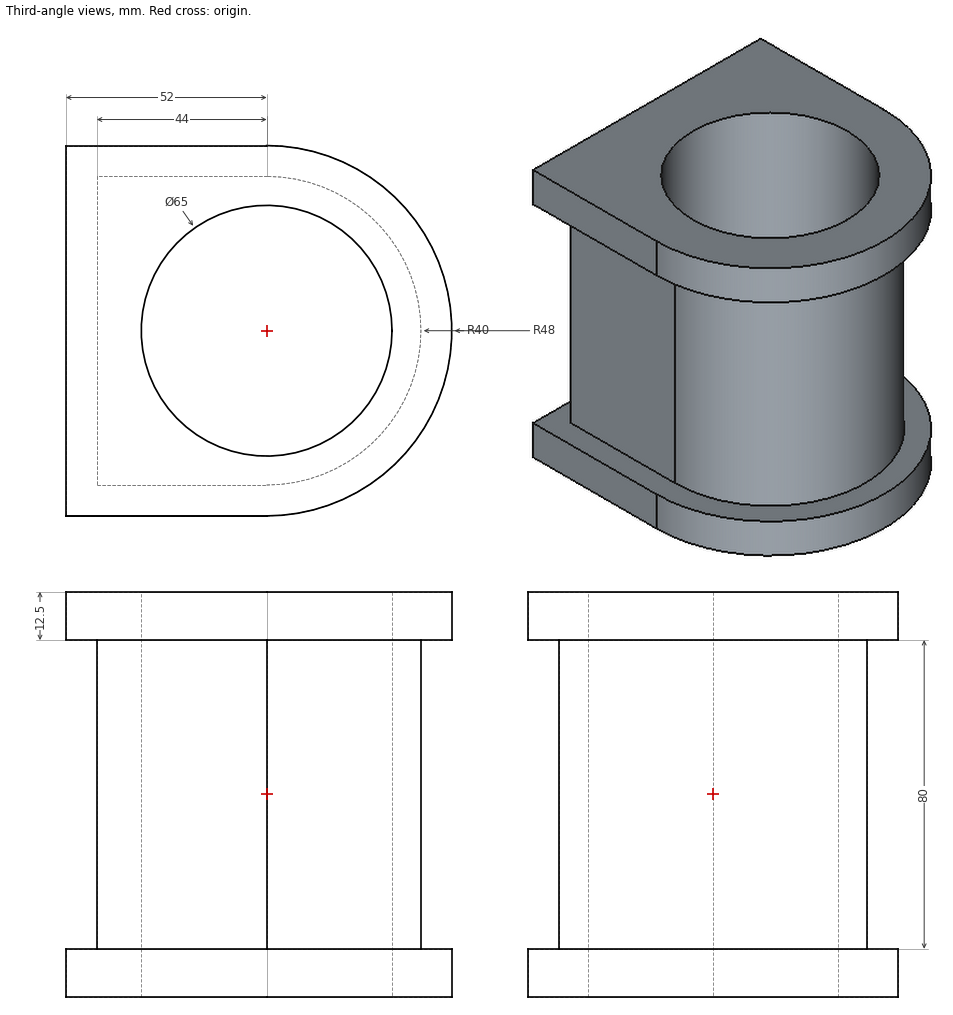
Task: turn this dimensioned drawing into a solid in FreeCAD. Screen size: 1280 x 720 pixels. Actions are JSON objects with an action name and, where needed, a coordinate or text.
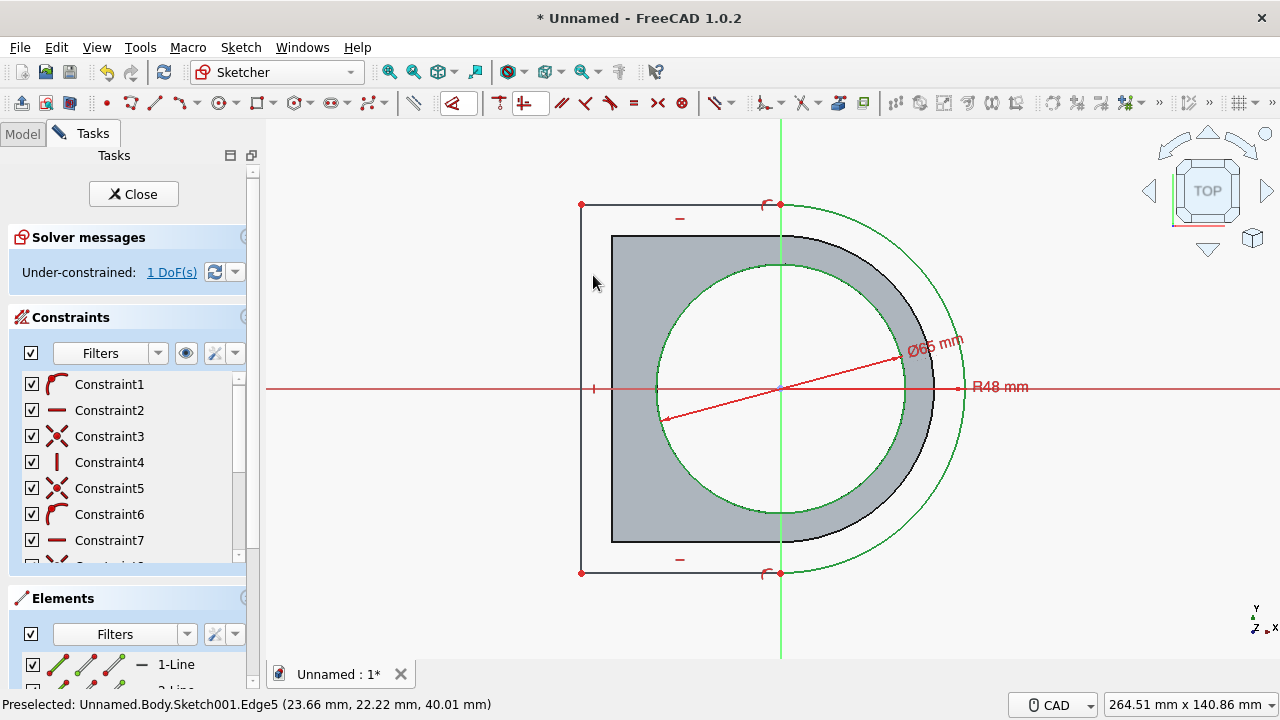
{"action": "left_click", "coordinate": [721, 205]}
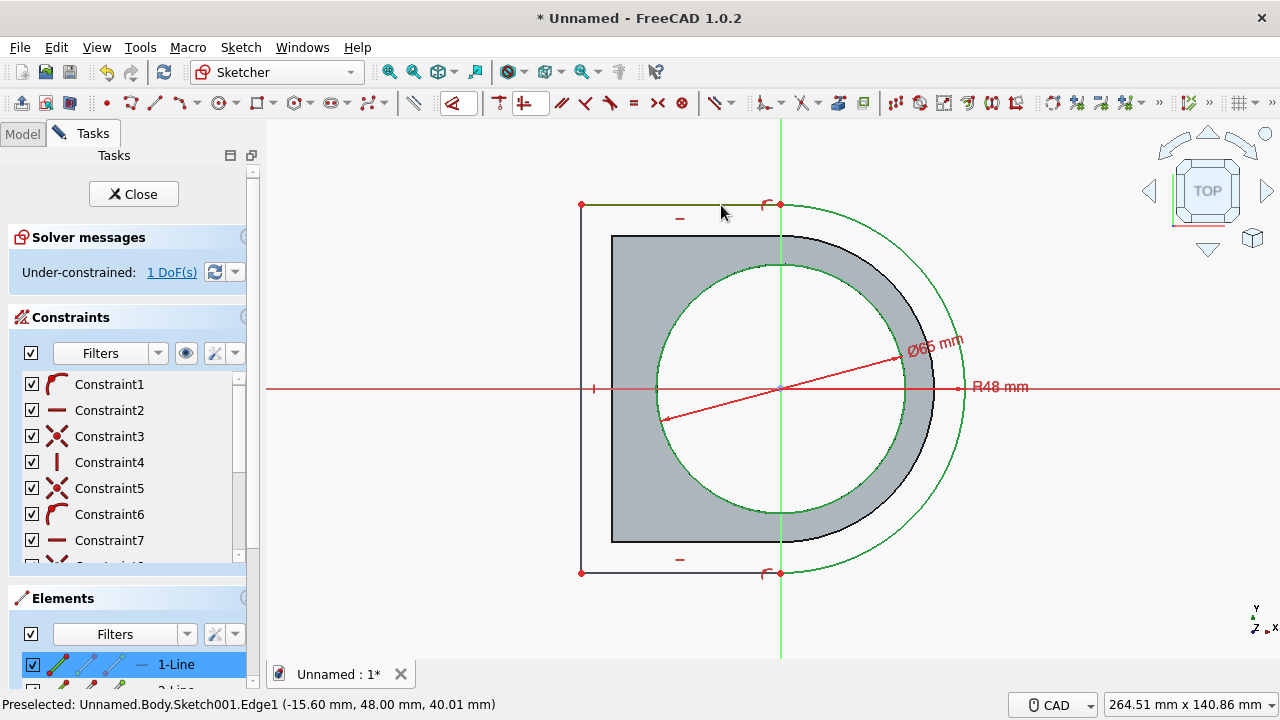
{"action": "key", "text": "l"}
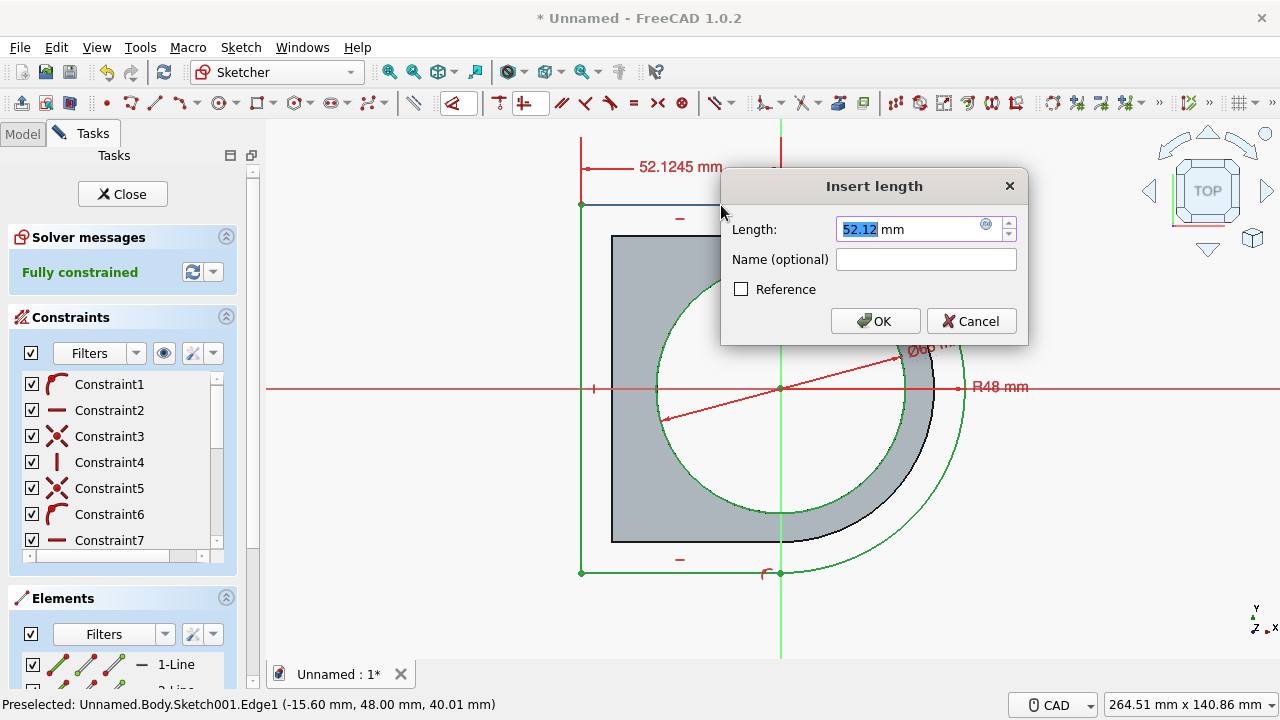
{"action": "type", "text": "52"}
{"action": "key", "text": "Return"}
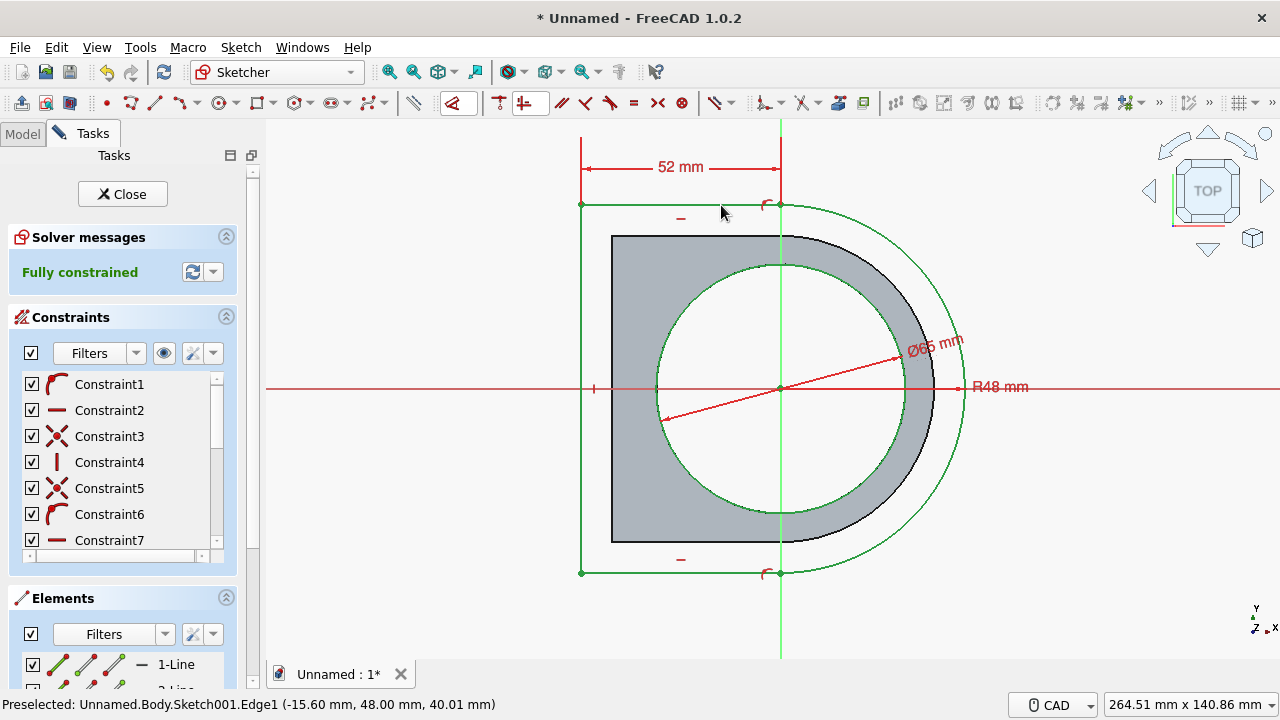
{"action": "left_click", "coordinate": [123, 194]}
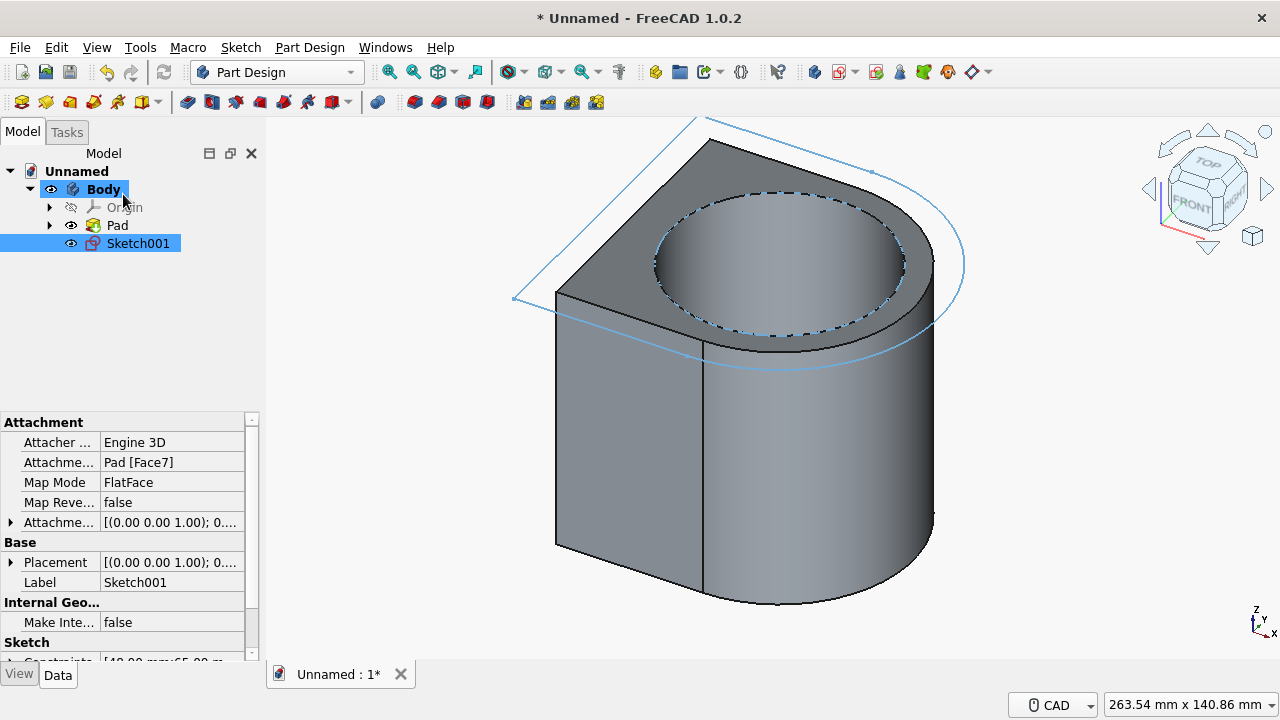
{"action": "left_click", "coordinate": [22, 102]}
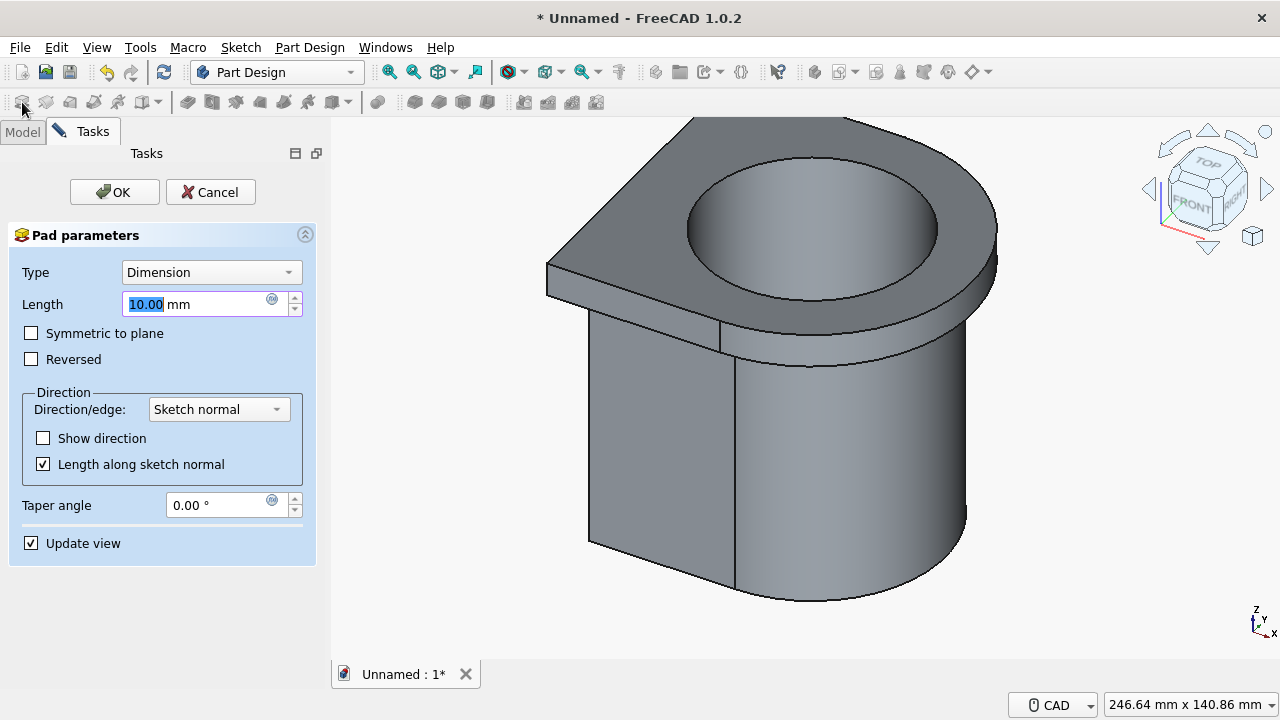
{"action": "type", "text": "12.5"}
{"action": "key", "text": "Tab"}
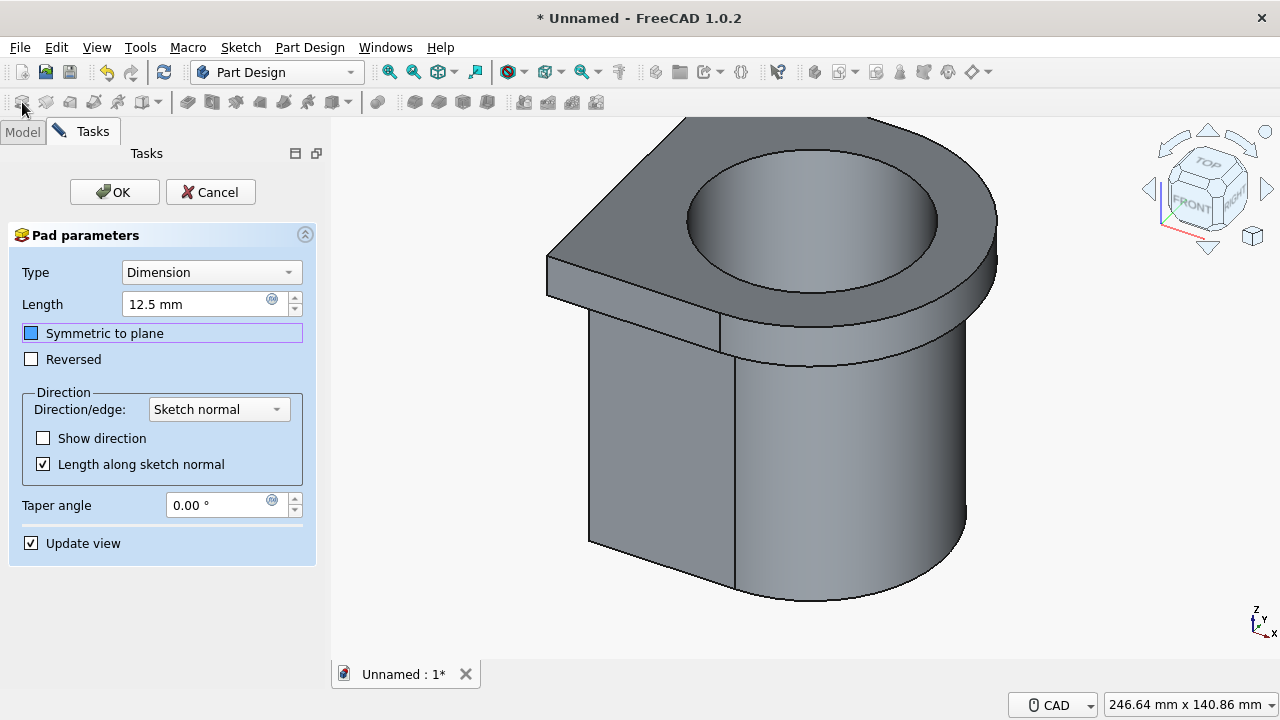
{"action": "left_click", "coordinate": [115, 192]}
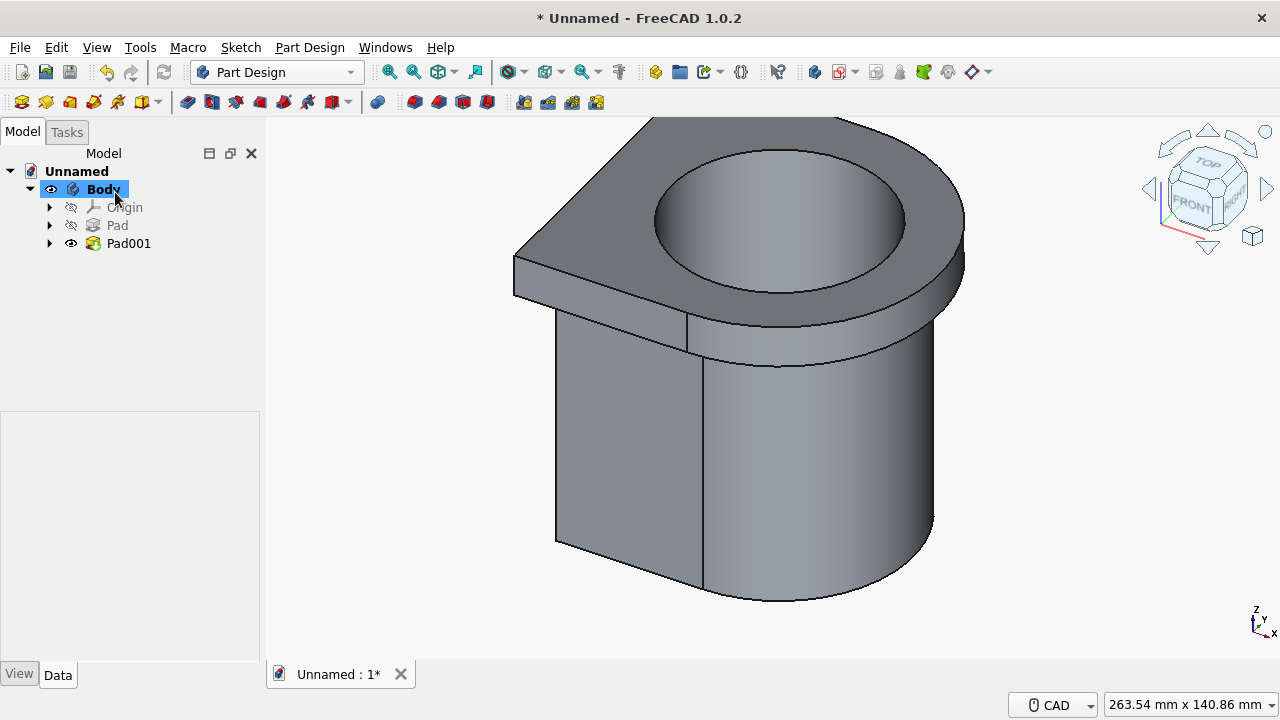
{"action": "left_click", "coordinate": [390, 72]}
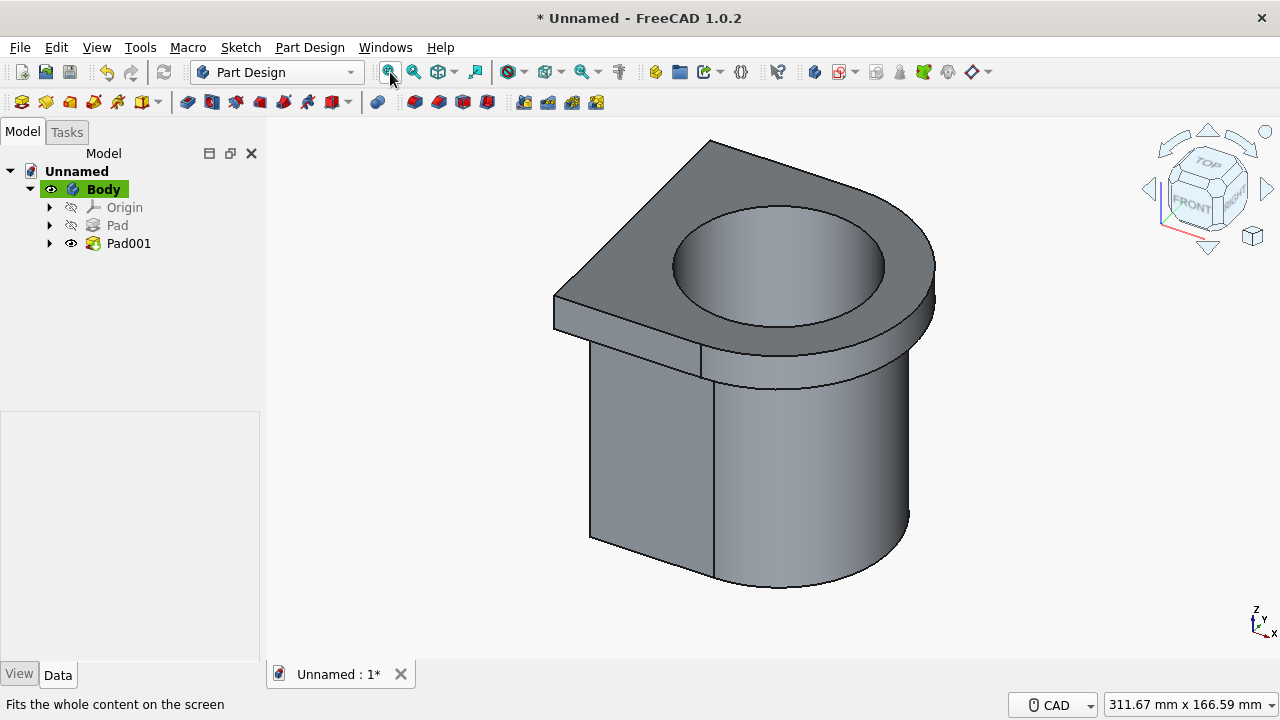
{"action": "left_click", "coordinate": [116, 243]}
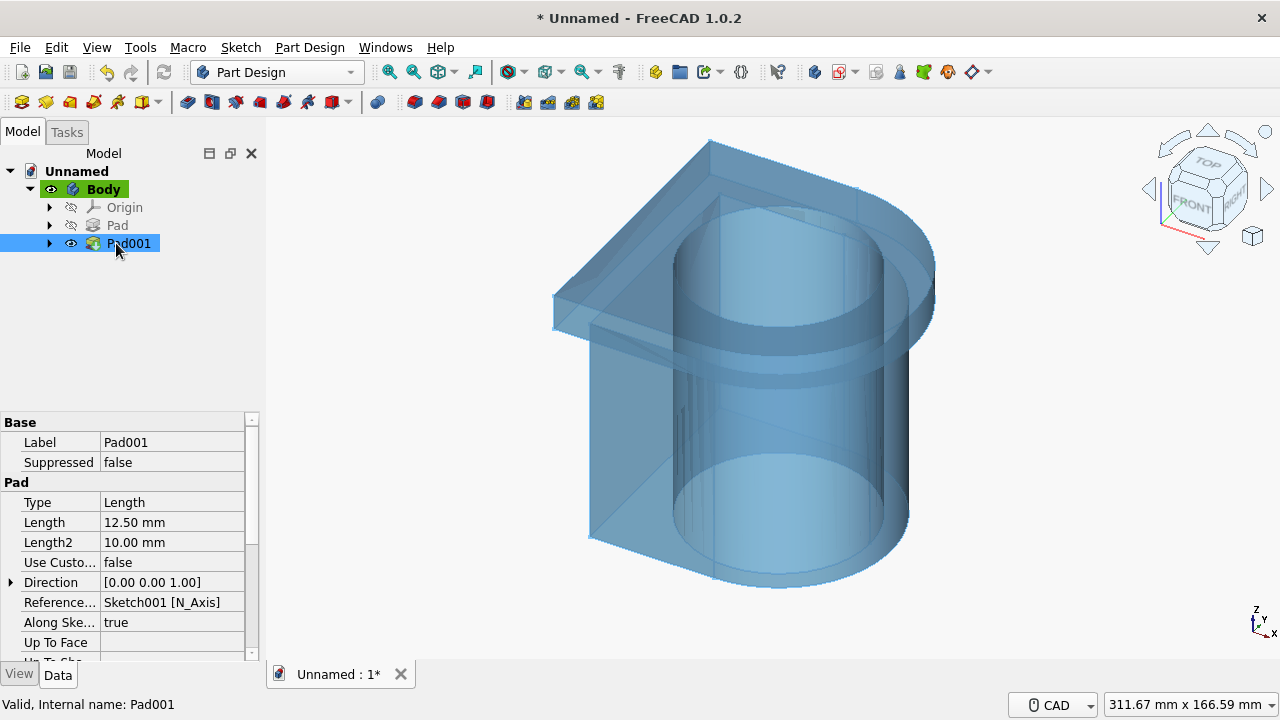
{"action": "left_click", "coordinate": [524, 102]}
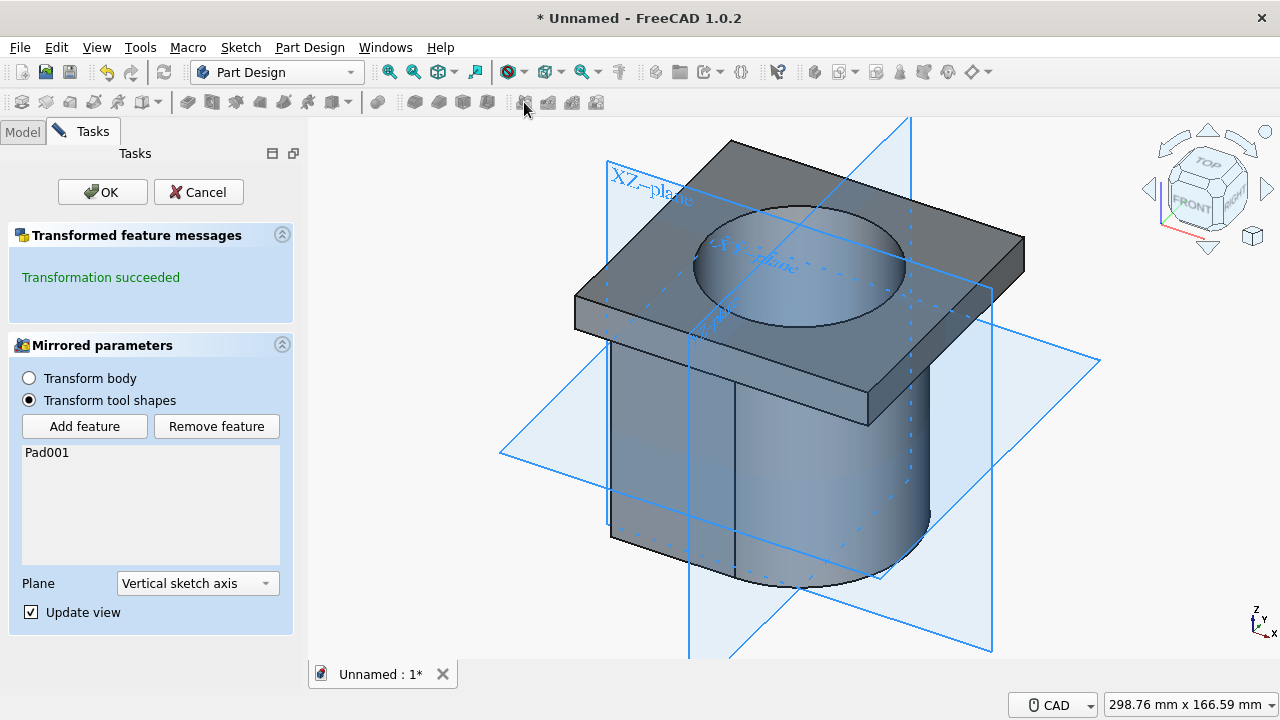
{"action": "left_click", "coordinate": [198, 584]}